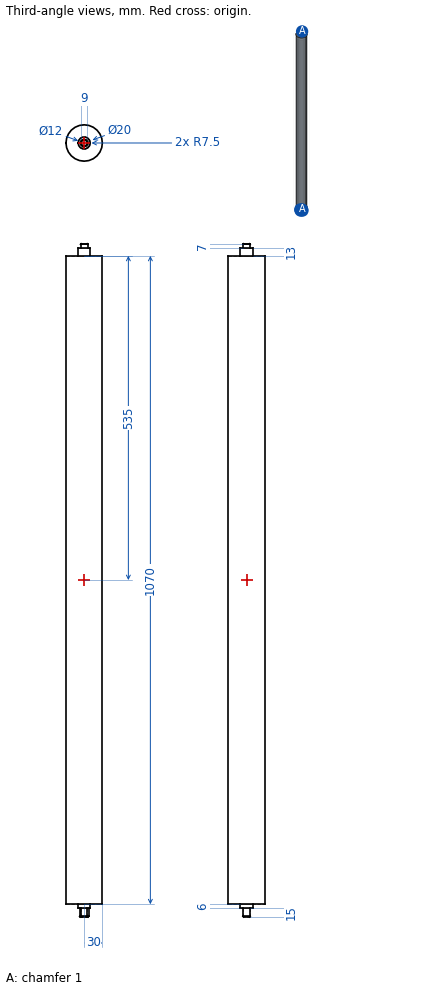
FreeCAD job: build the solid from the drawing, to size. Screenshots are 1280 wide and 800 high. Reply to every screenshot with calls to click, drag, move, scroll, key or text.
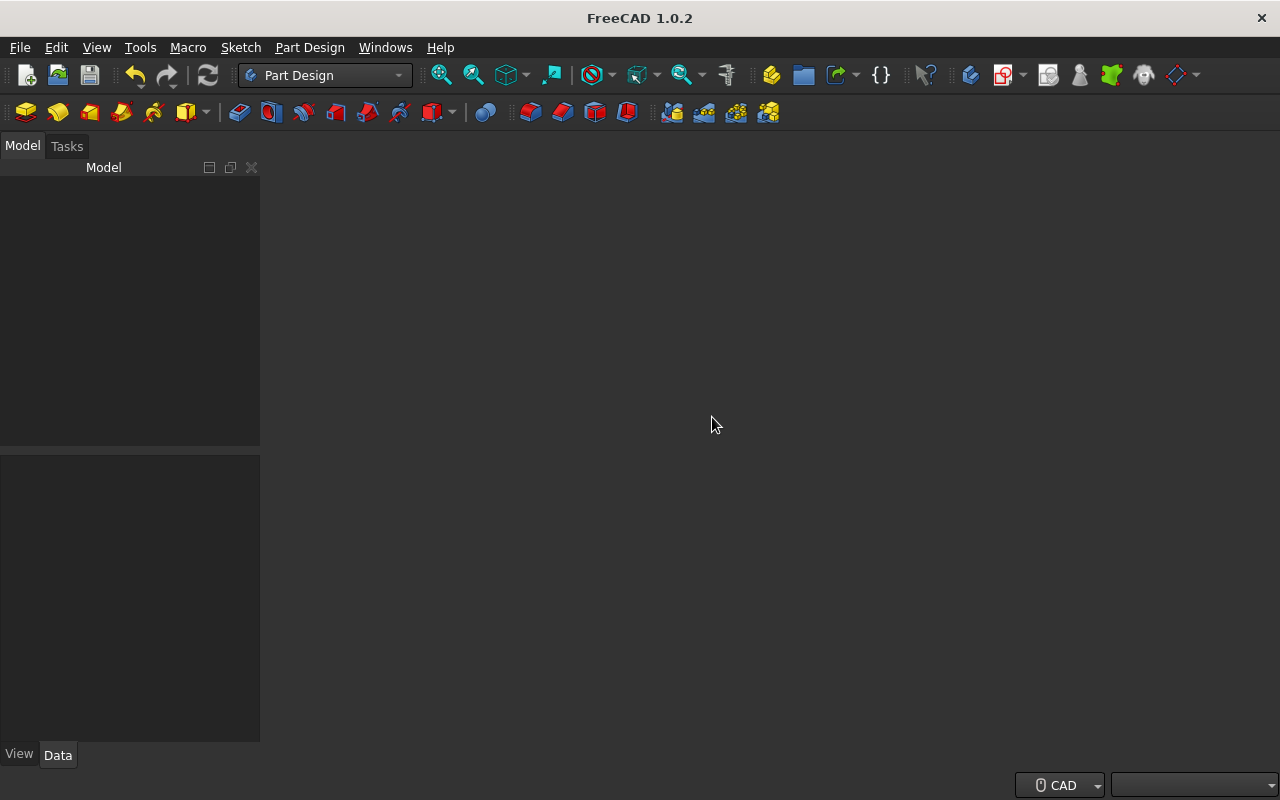
click(26, 76)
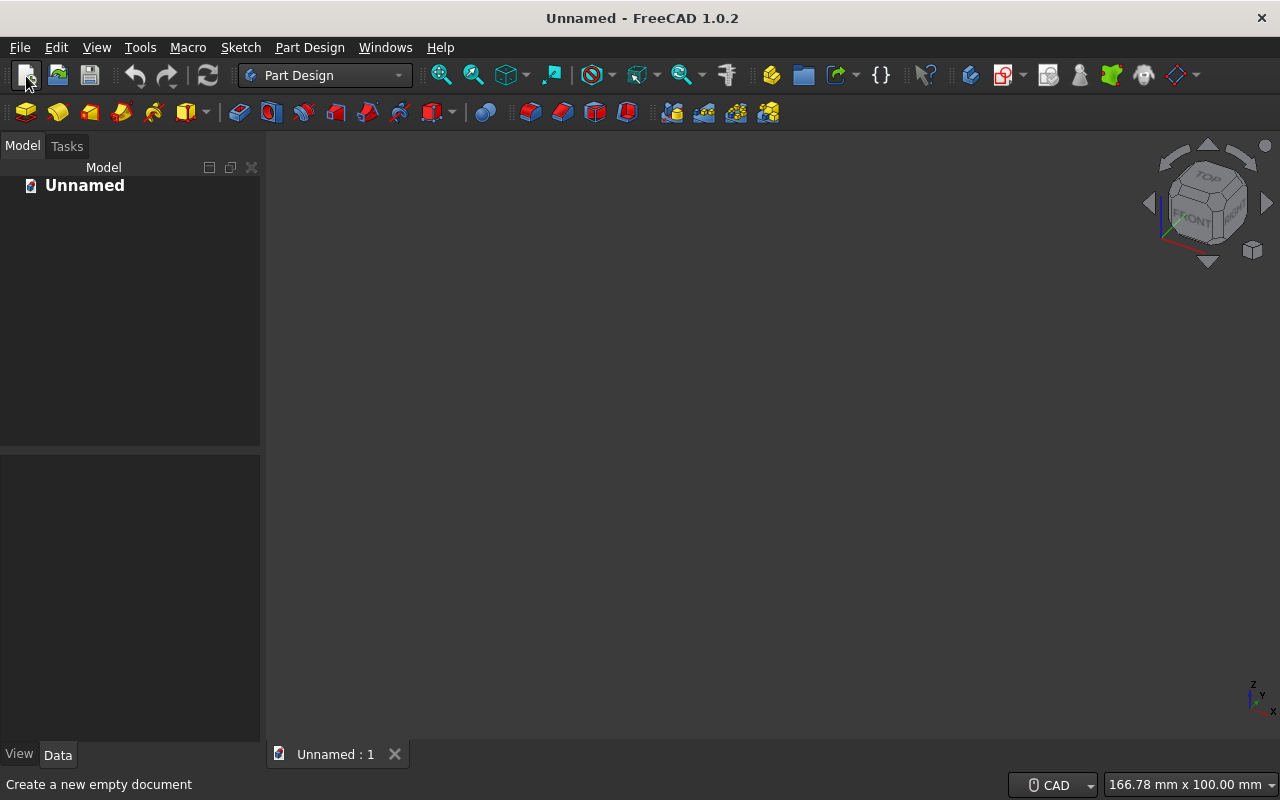
click(1004, 76)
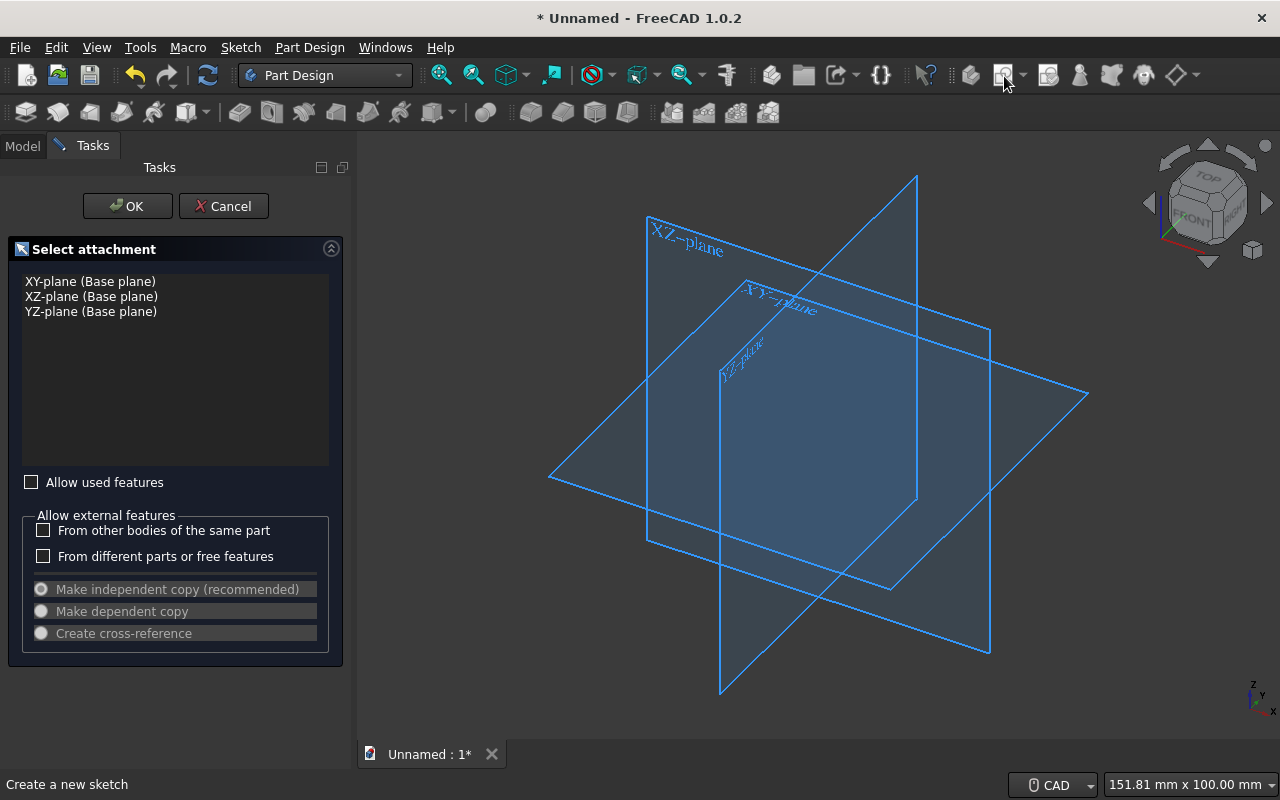
click(82, 296)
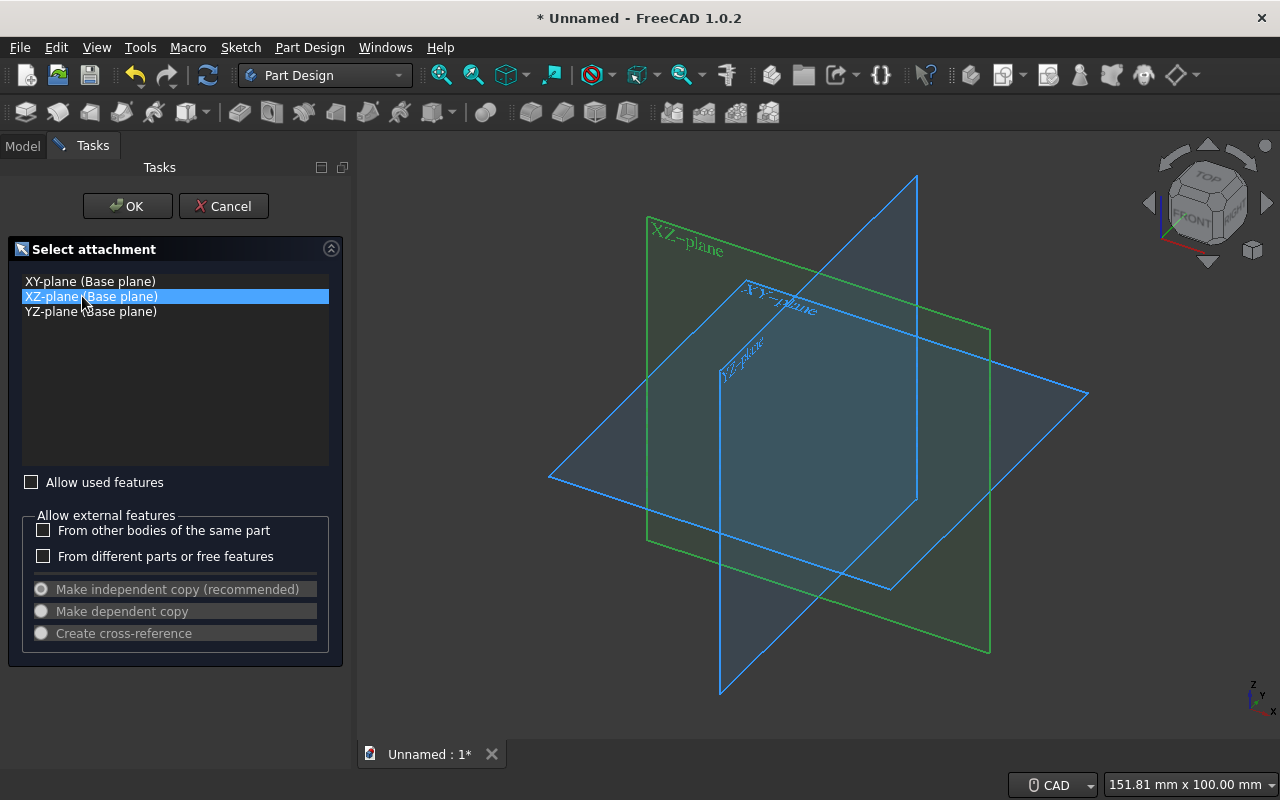
click(128, 206)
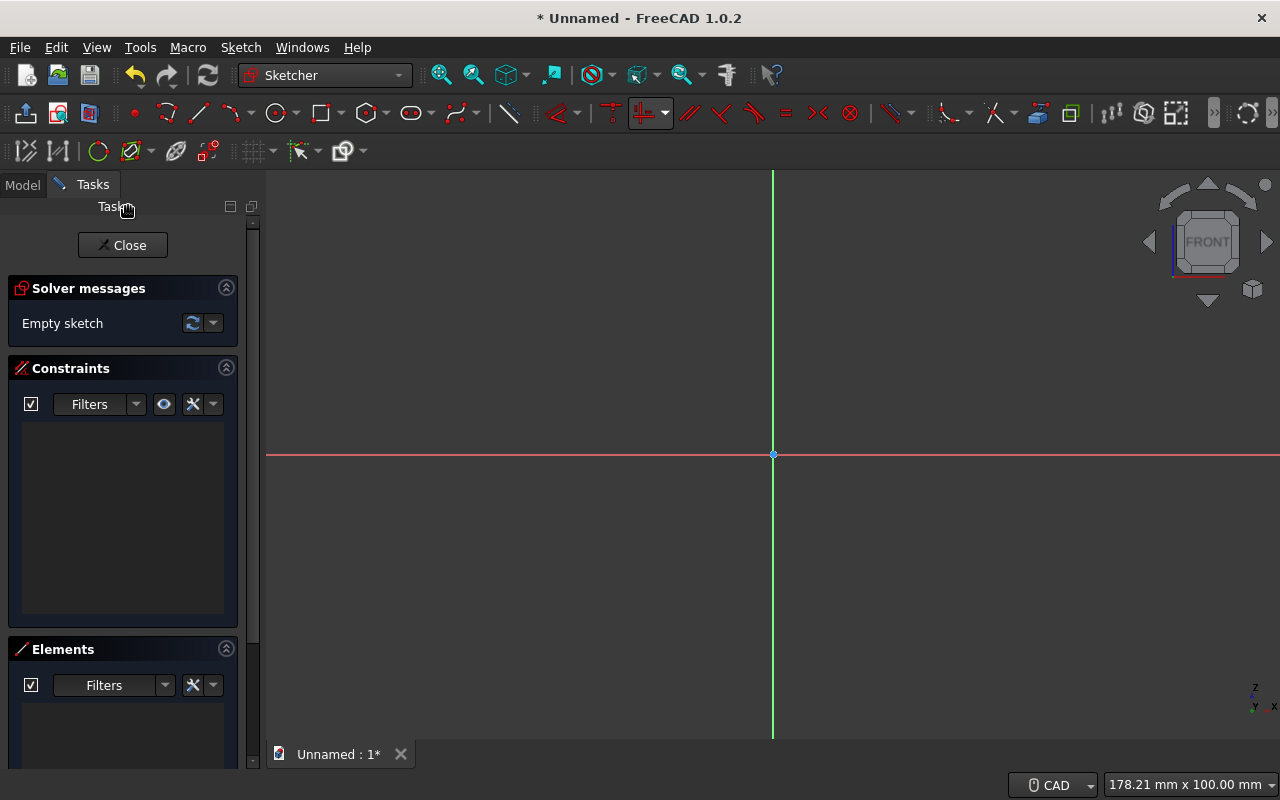
scroll(695, 454, down, 14)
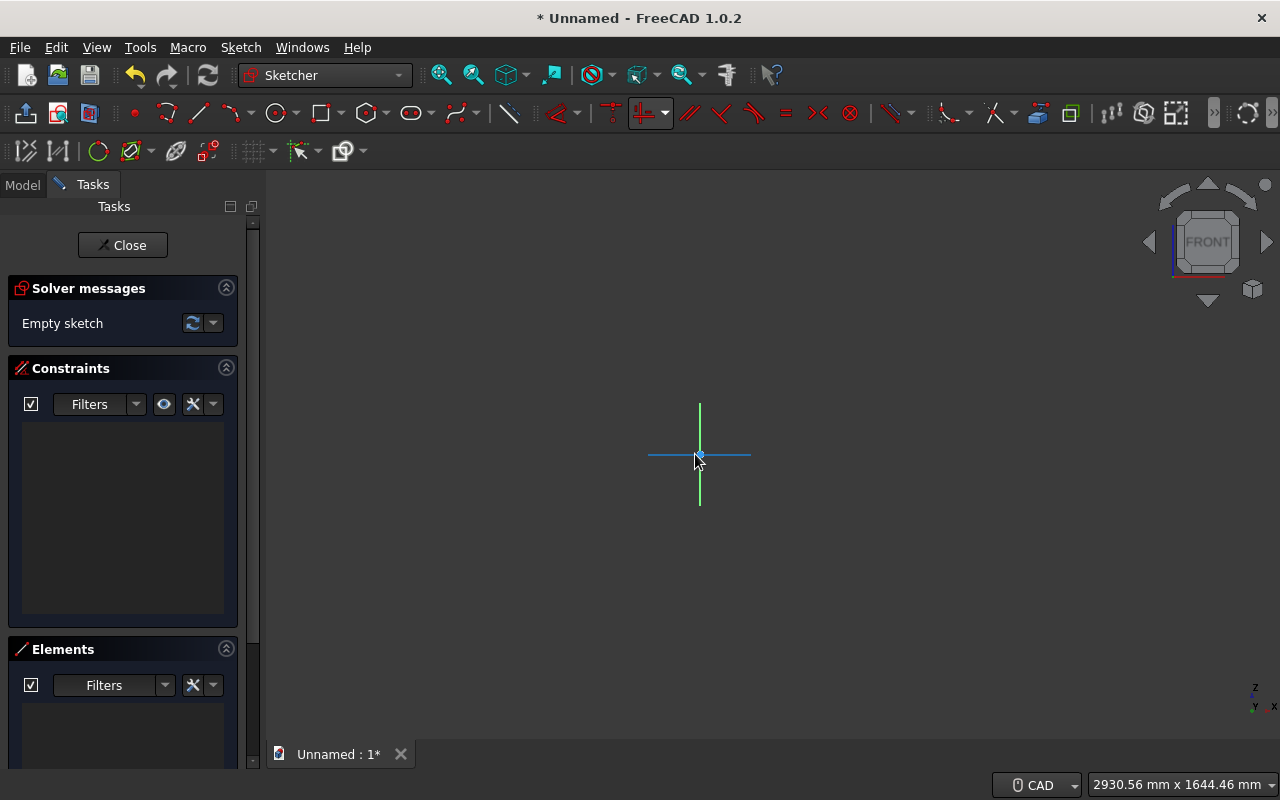
key(g)
key(r)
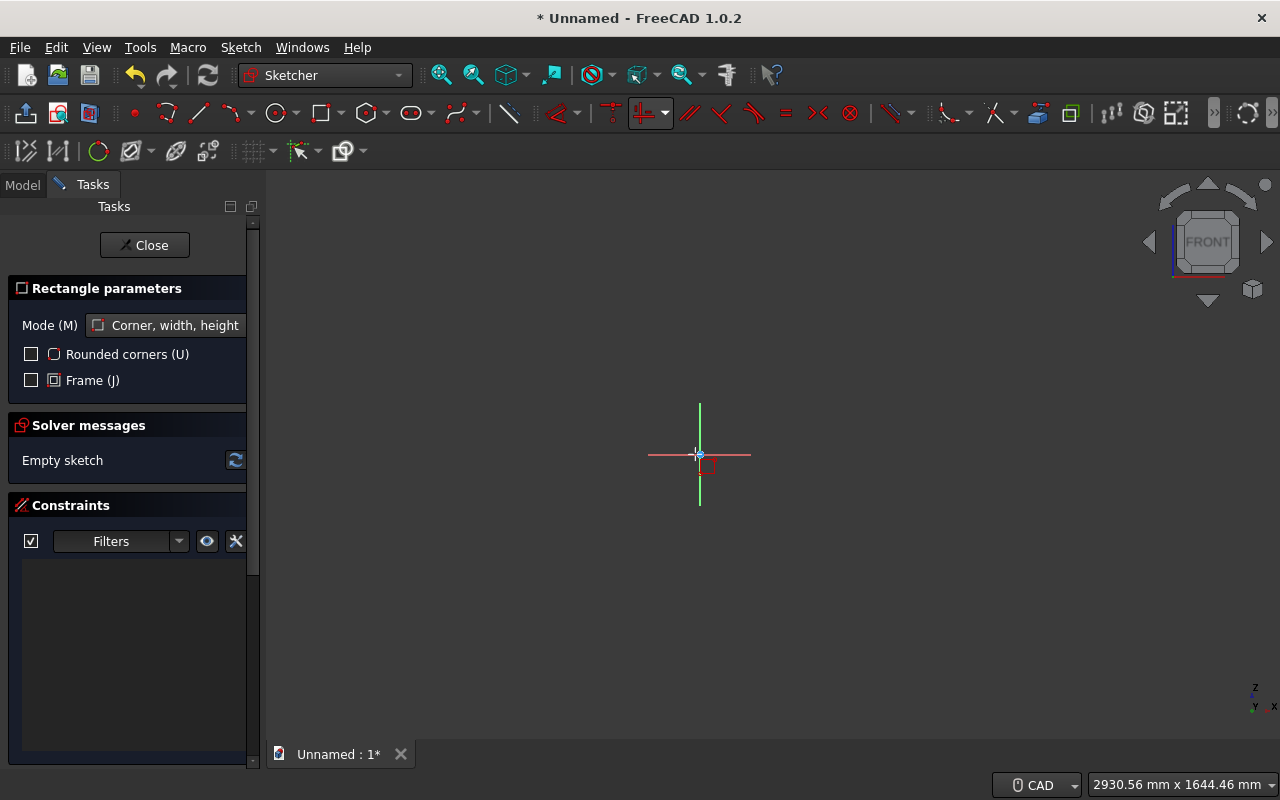
scroll(700, 269, up, 3)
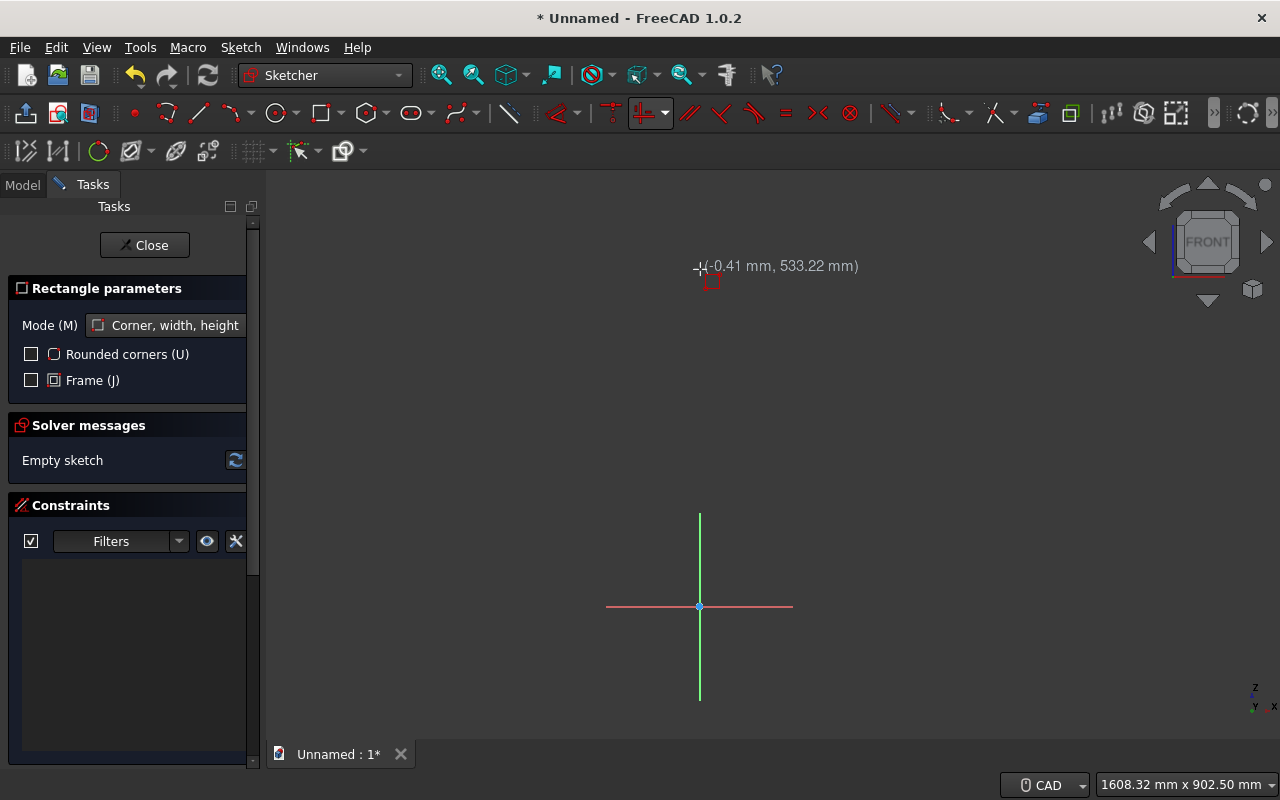
click(700, 270)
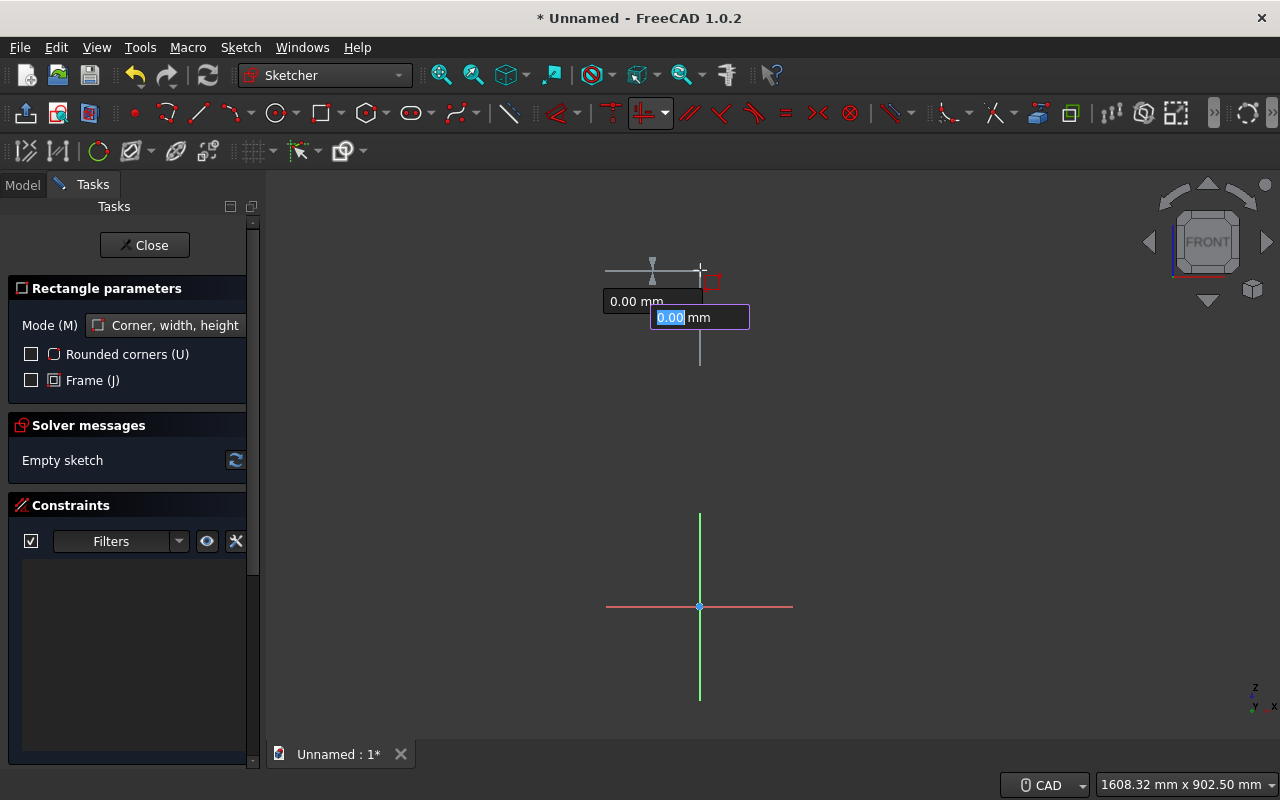
scroll(699, 269, down, 3)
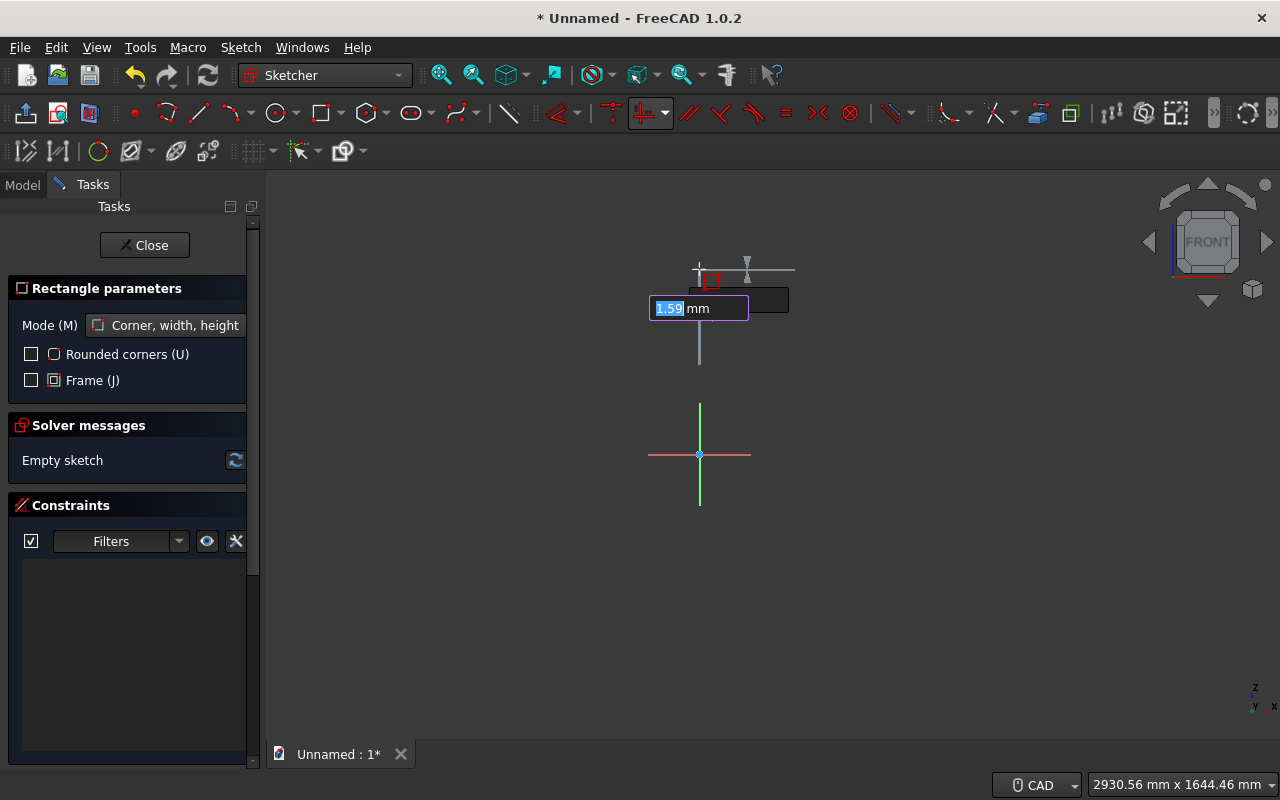
scroll(710, 640, up, 3)